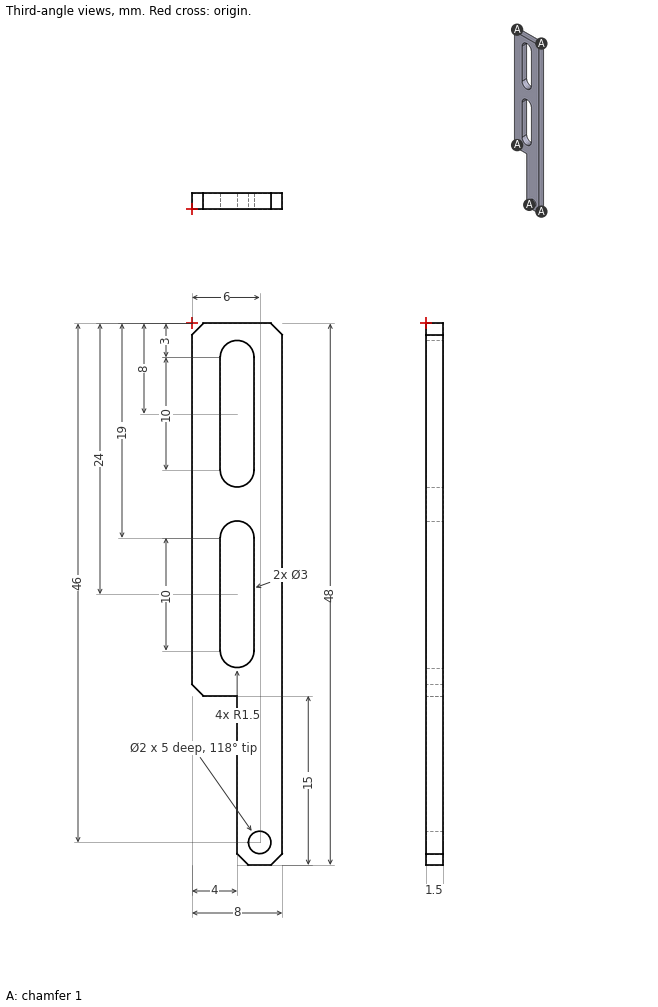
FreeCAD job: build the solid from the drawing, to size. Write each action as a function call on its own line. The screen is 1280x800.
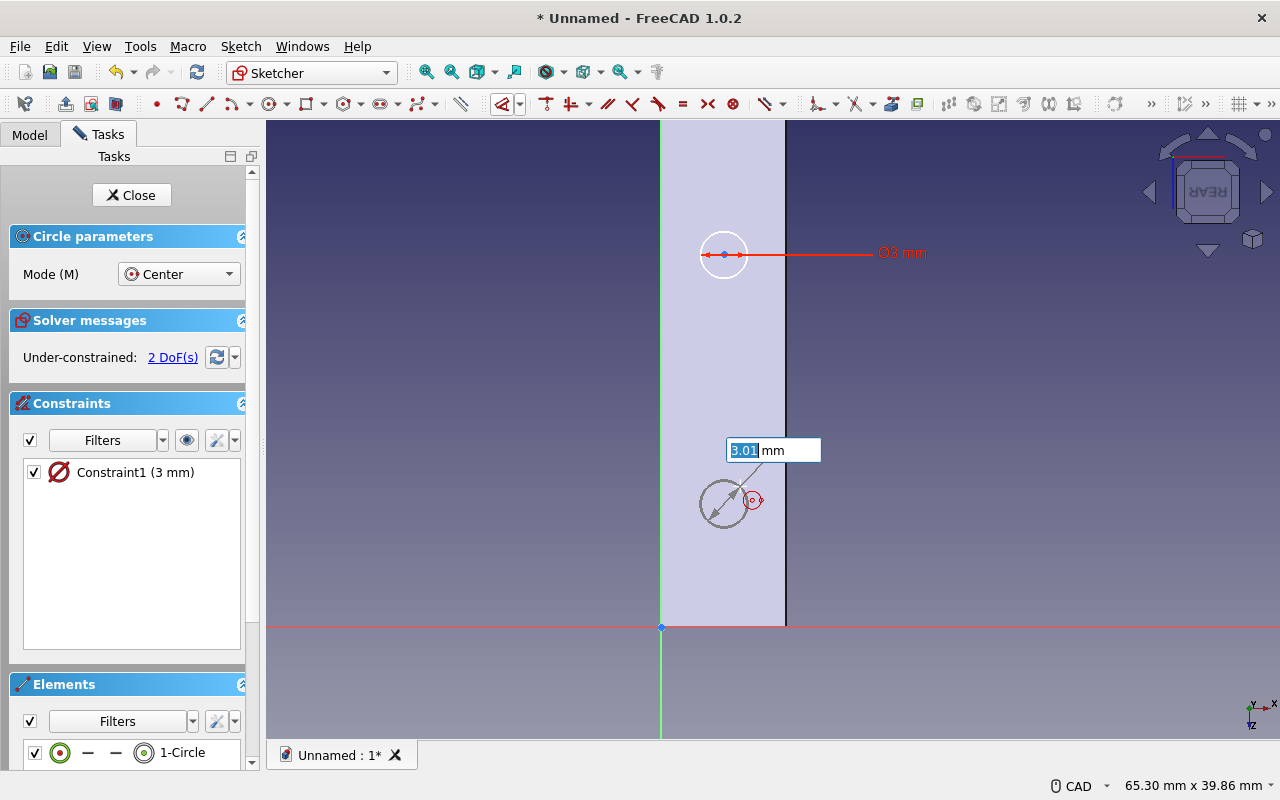
text(3)
key(Return)
key(Escape)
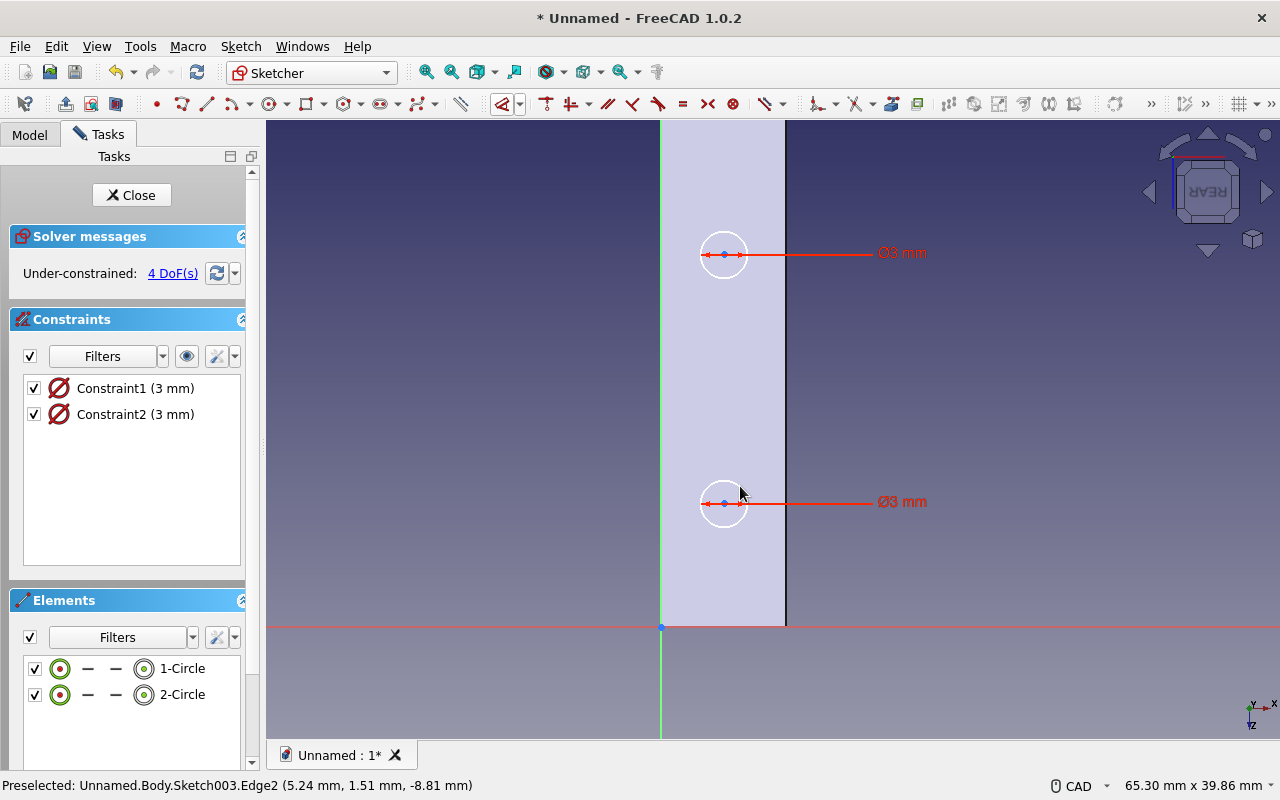
click(724, 255)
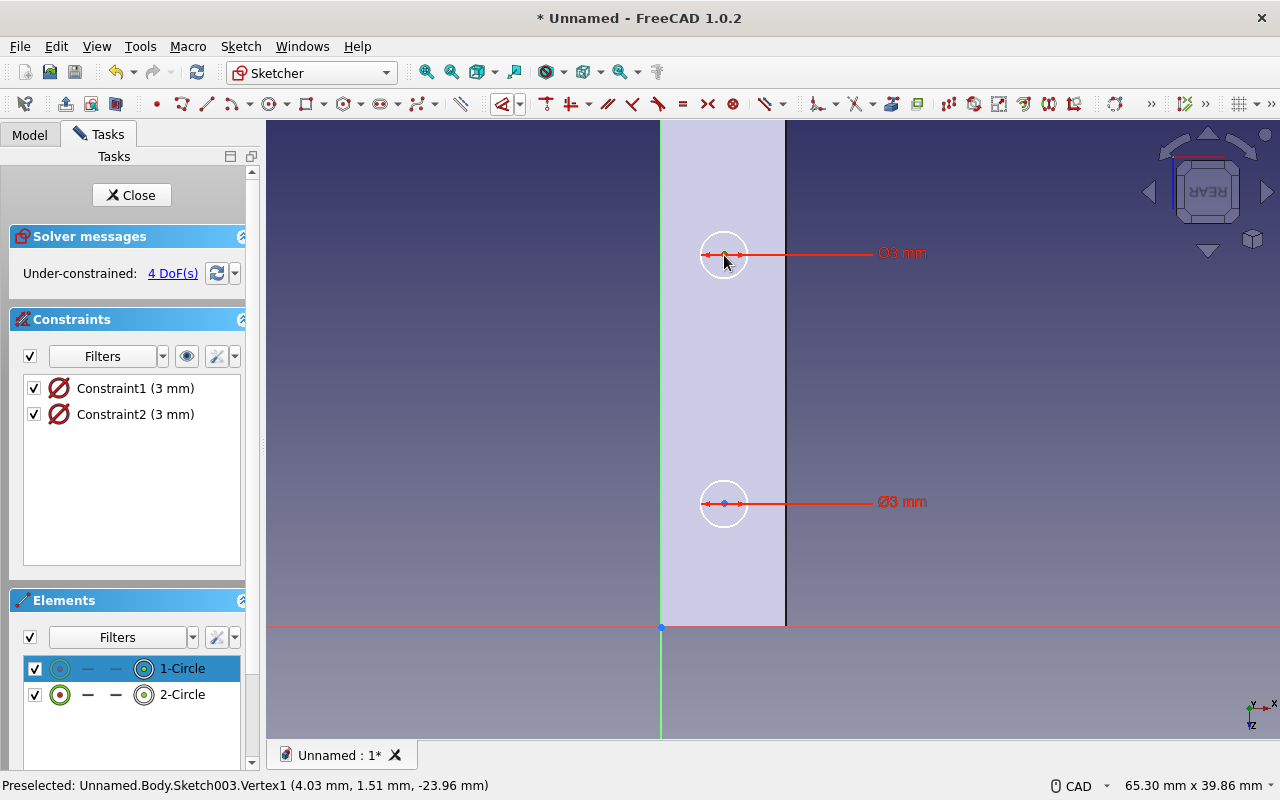
click(724, 504)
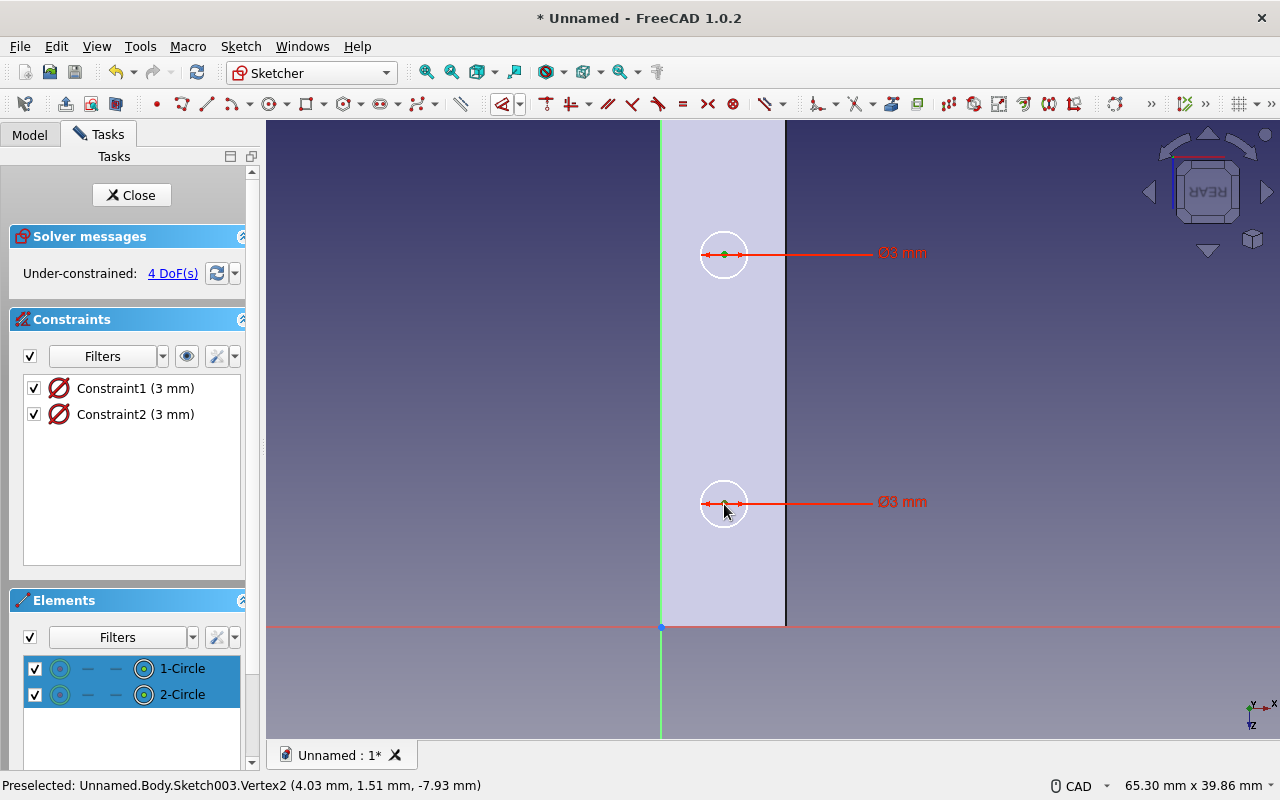
key(v)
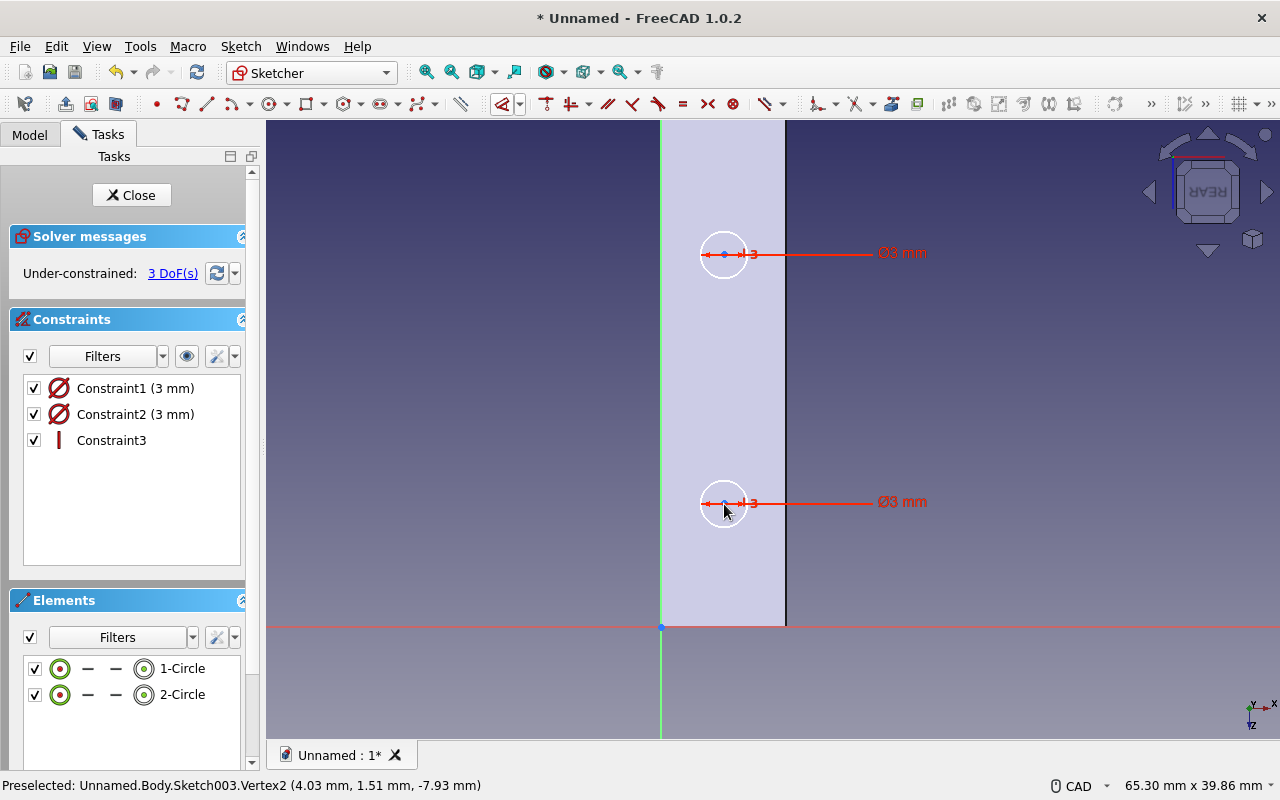
click(724, 255)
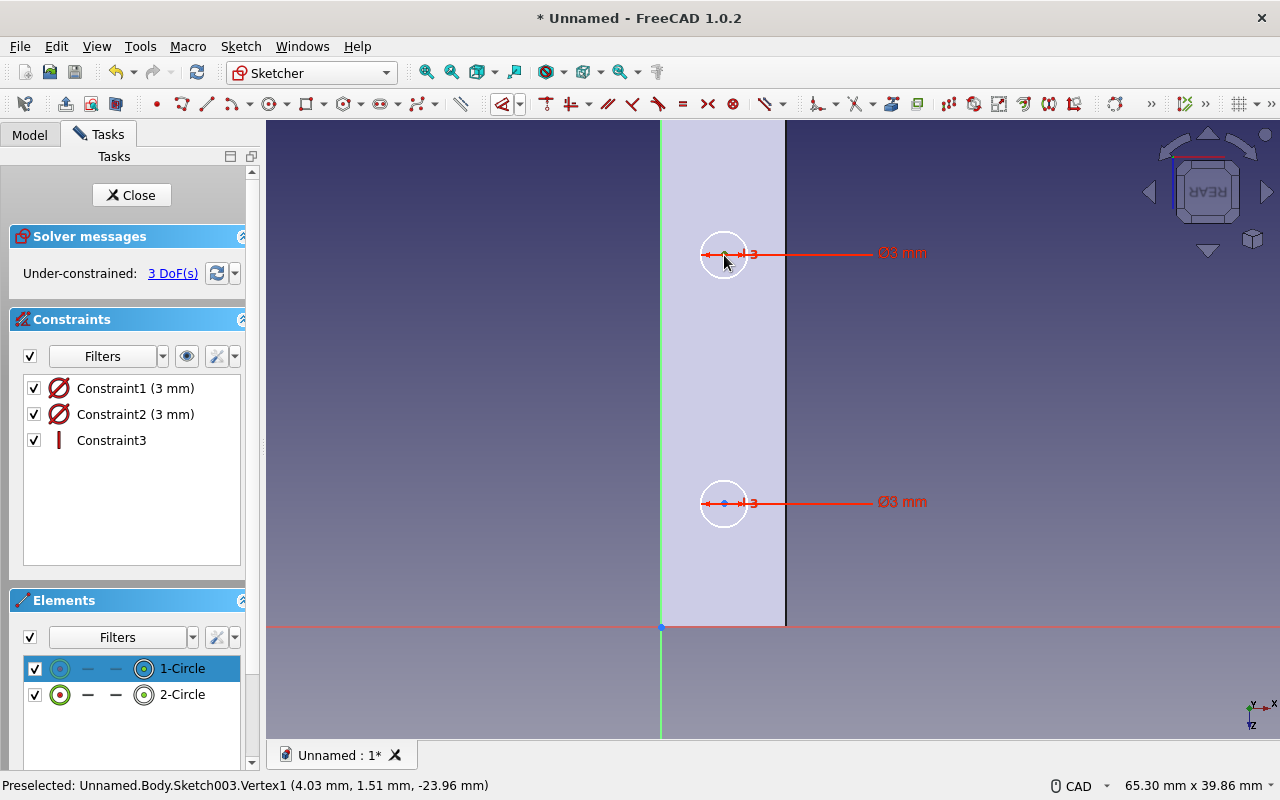
click(520, 104)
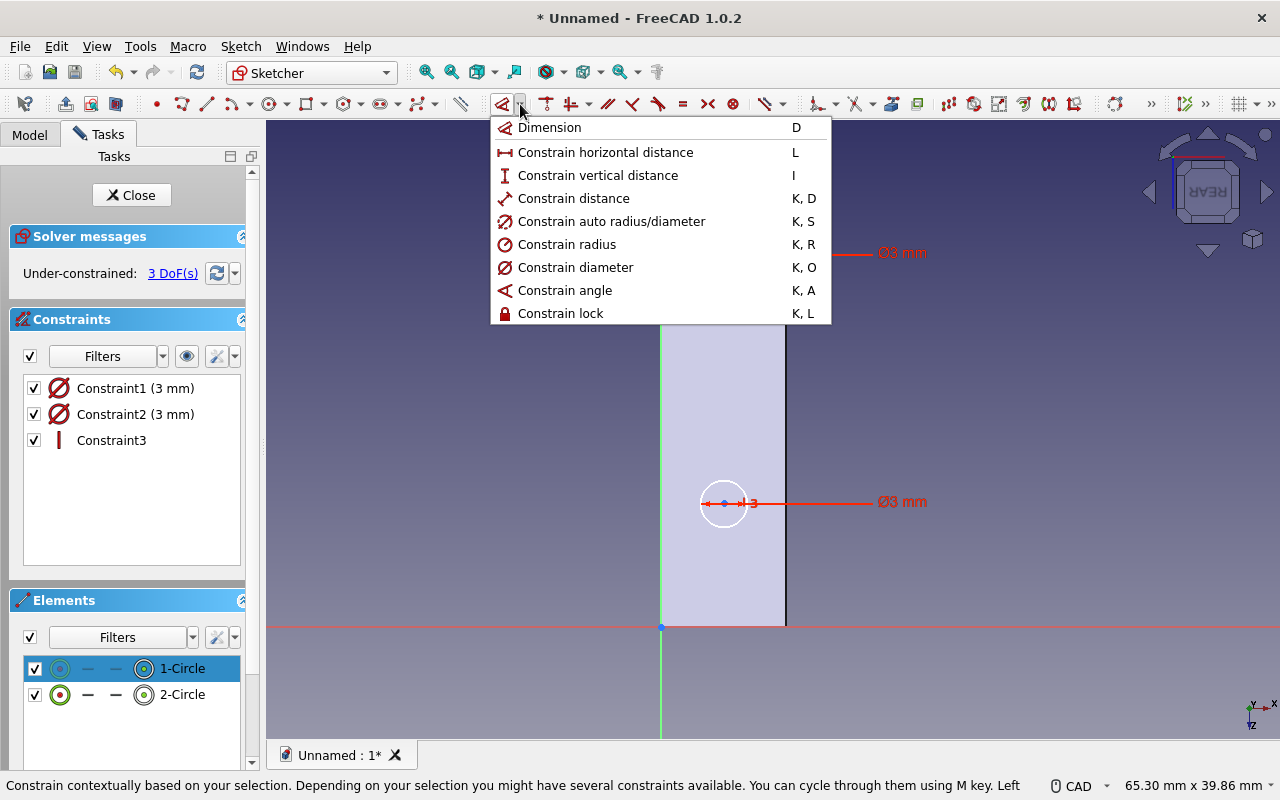
click(661, 152)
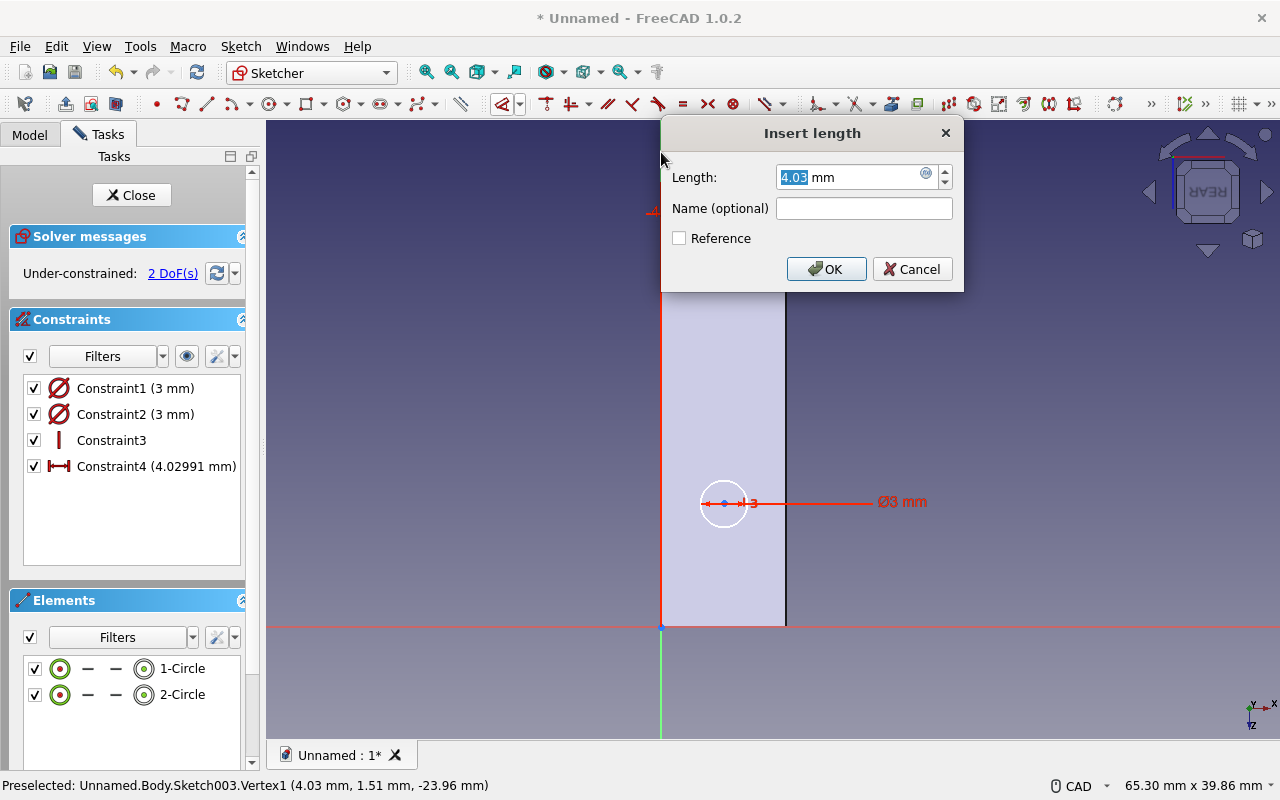
text(4)
key(Return)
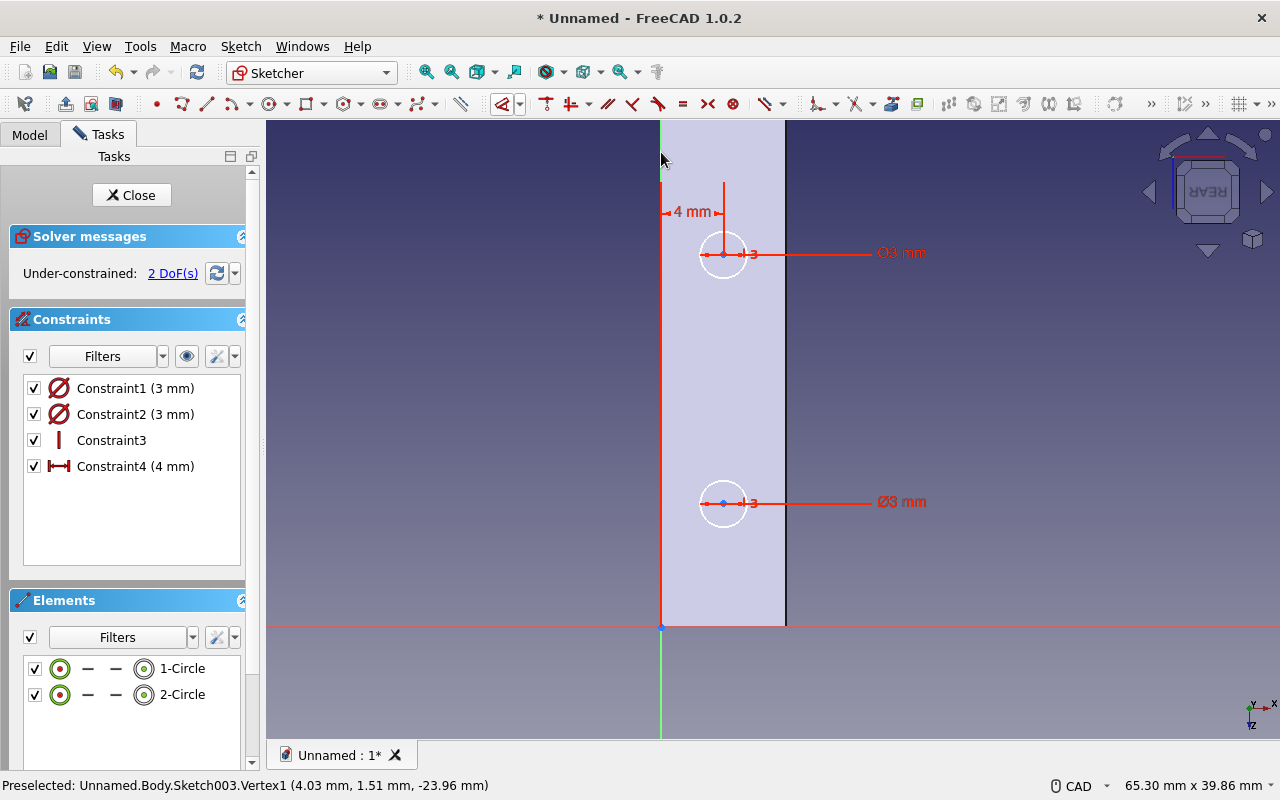
click(724, 504)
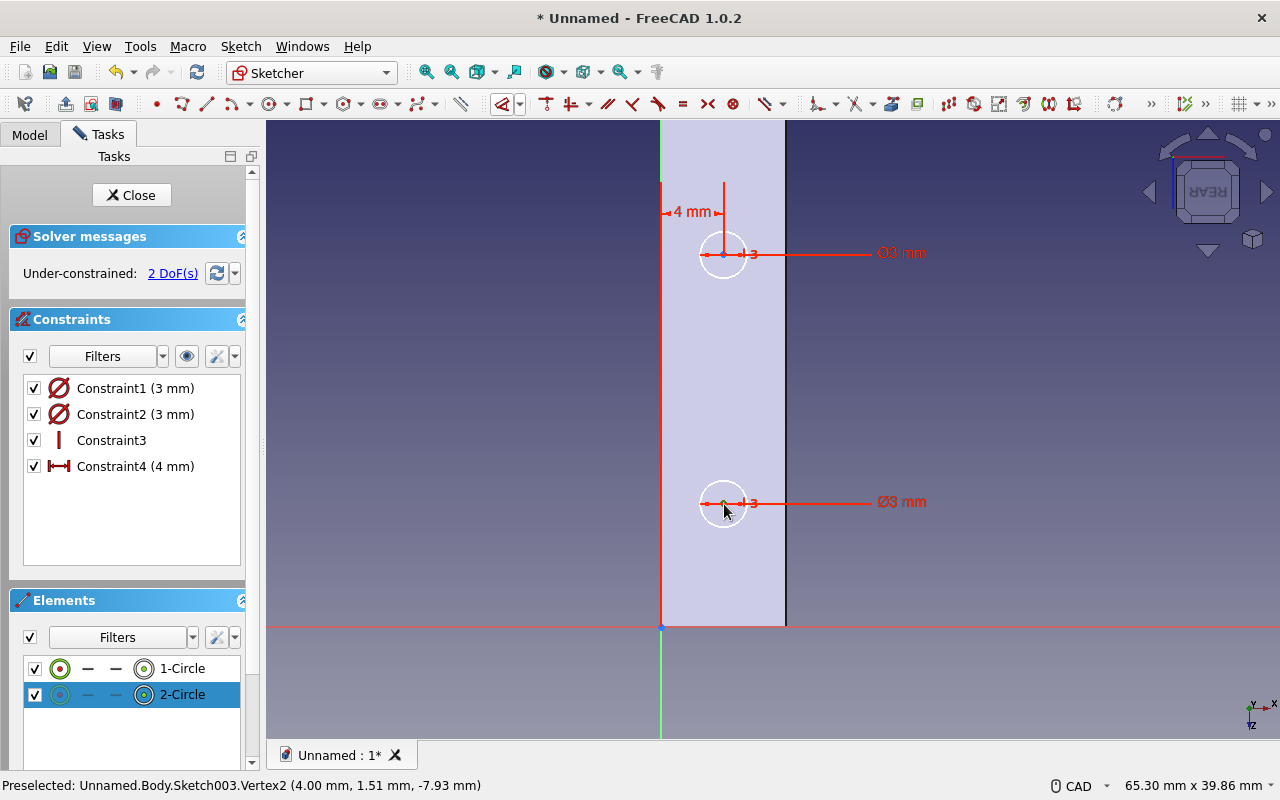
click(520, 104)